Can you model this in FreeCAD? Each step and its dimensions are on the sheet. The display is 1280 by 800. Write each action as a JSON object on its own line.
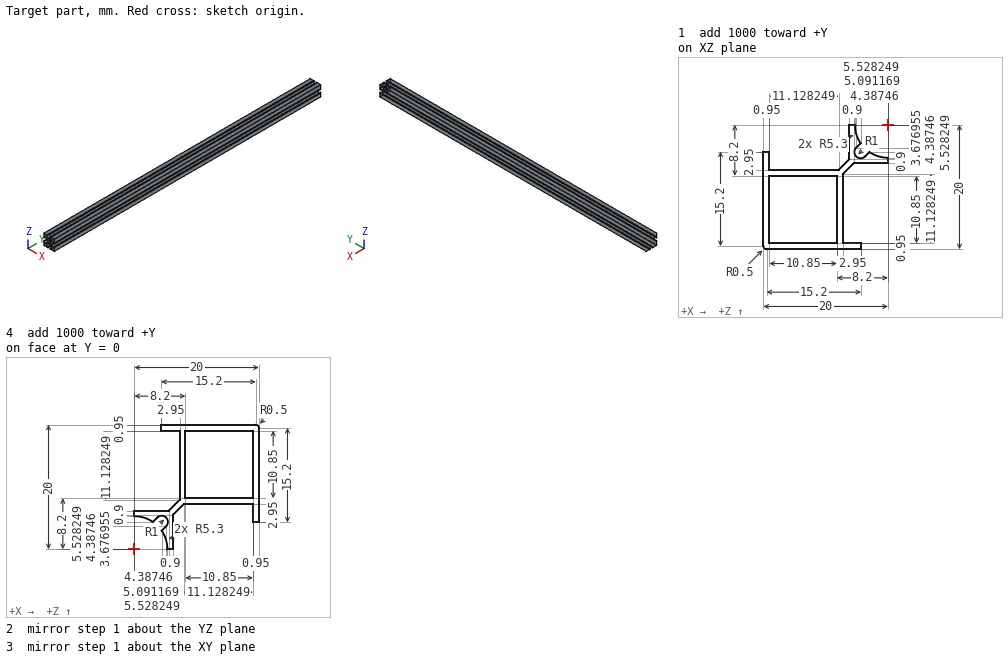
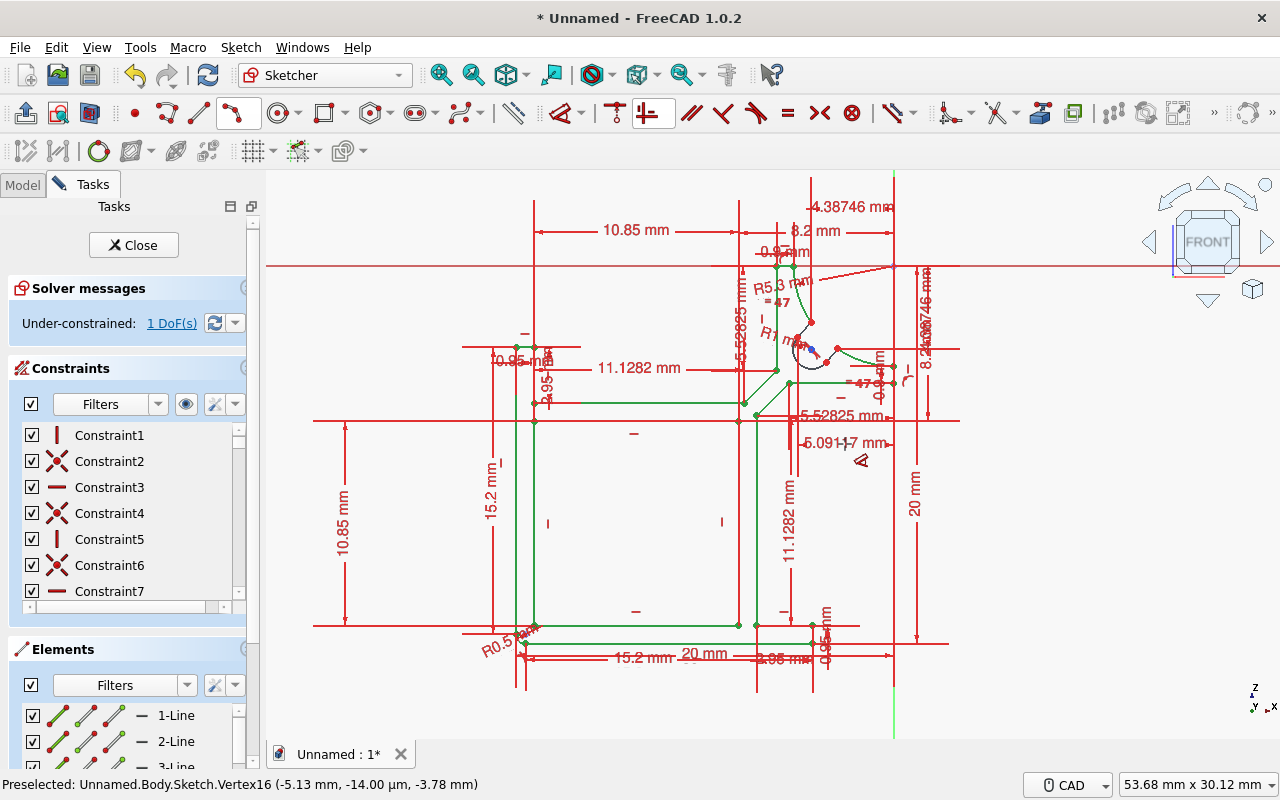
{"action": "left_click", "coordinate": [798, 338]}
{"action": "left_click", "coordinate": [928, 285]}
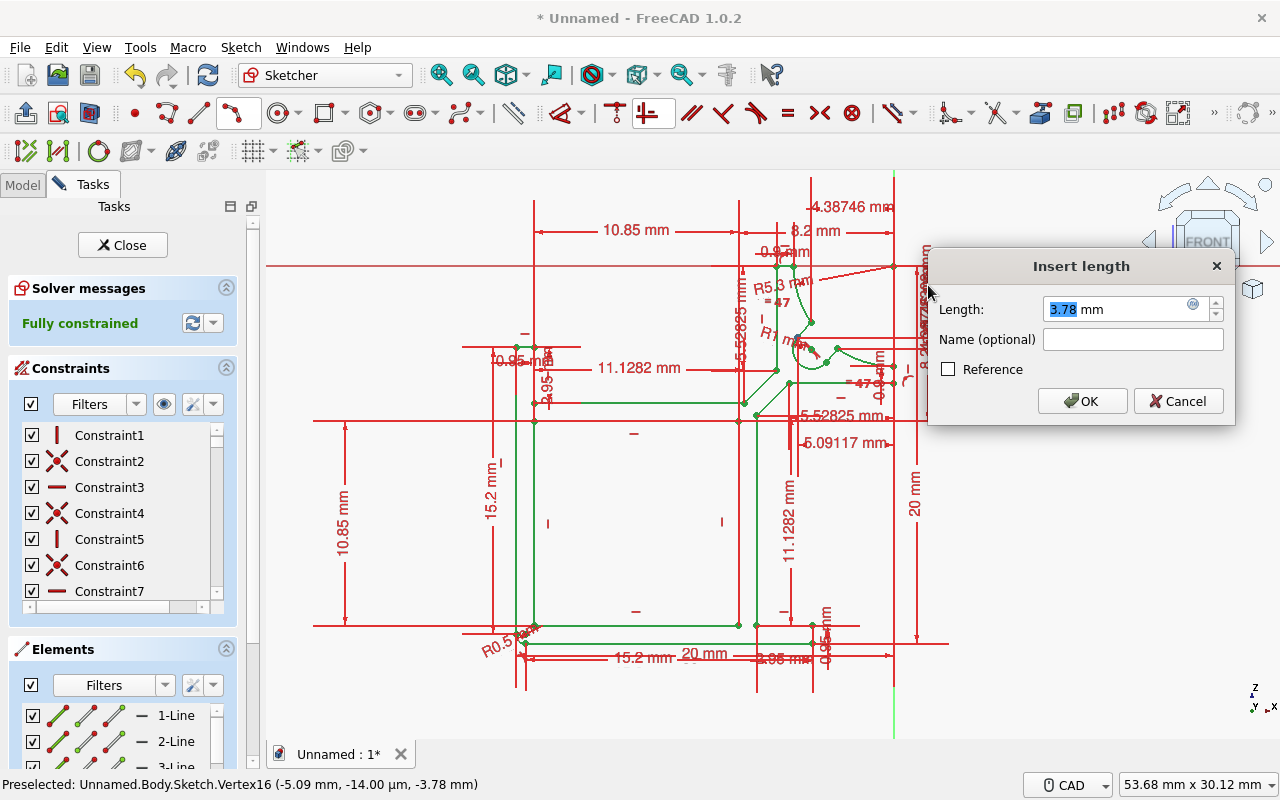
{"action": "type", "text": "3.676955"}
{"action": "key", "text": "Return"}
{"action": "key", "text": "Escape"}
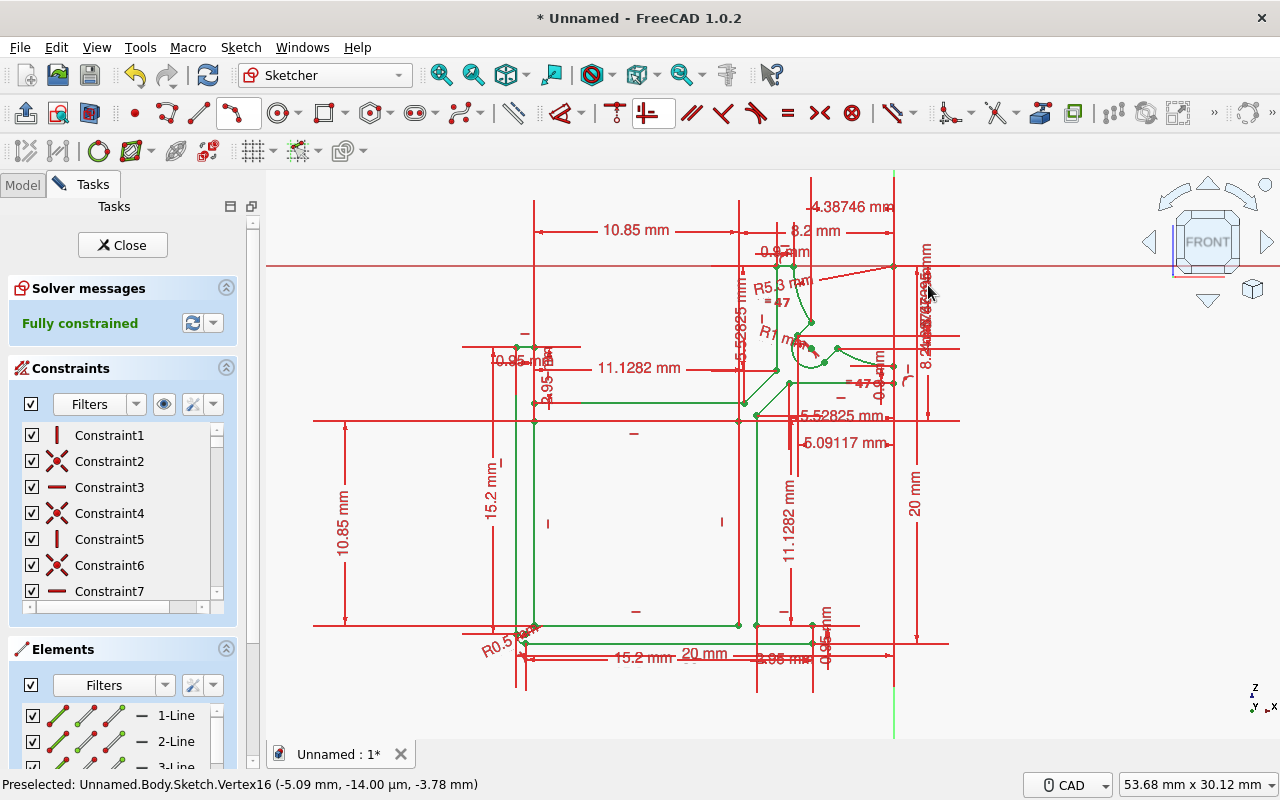
{"action": "left_click", "coordinate": [123, 245]}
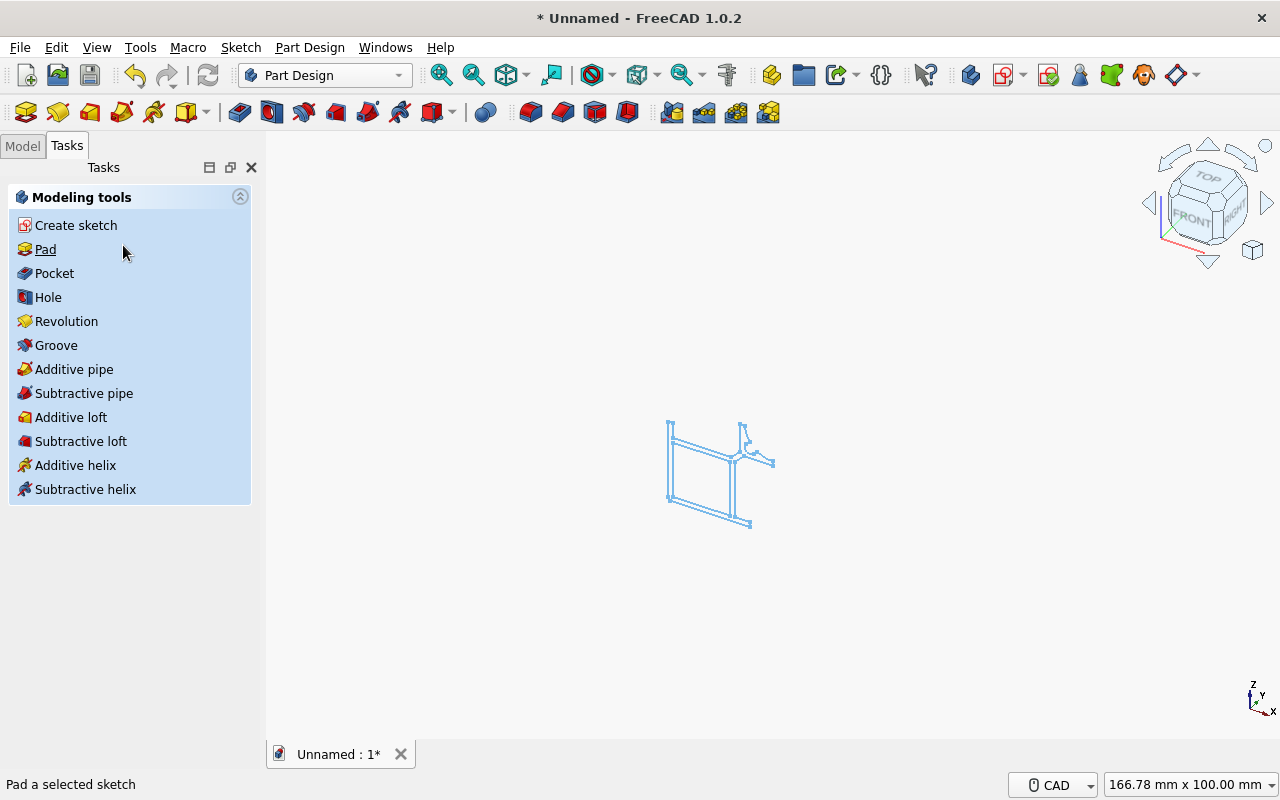
{"action": "left_click", "coordinate": [26, 112]}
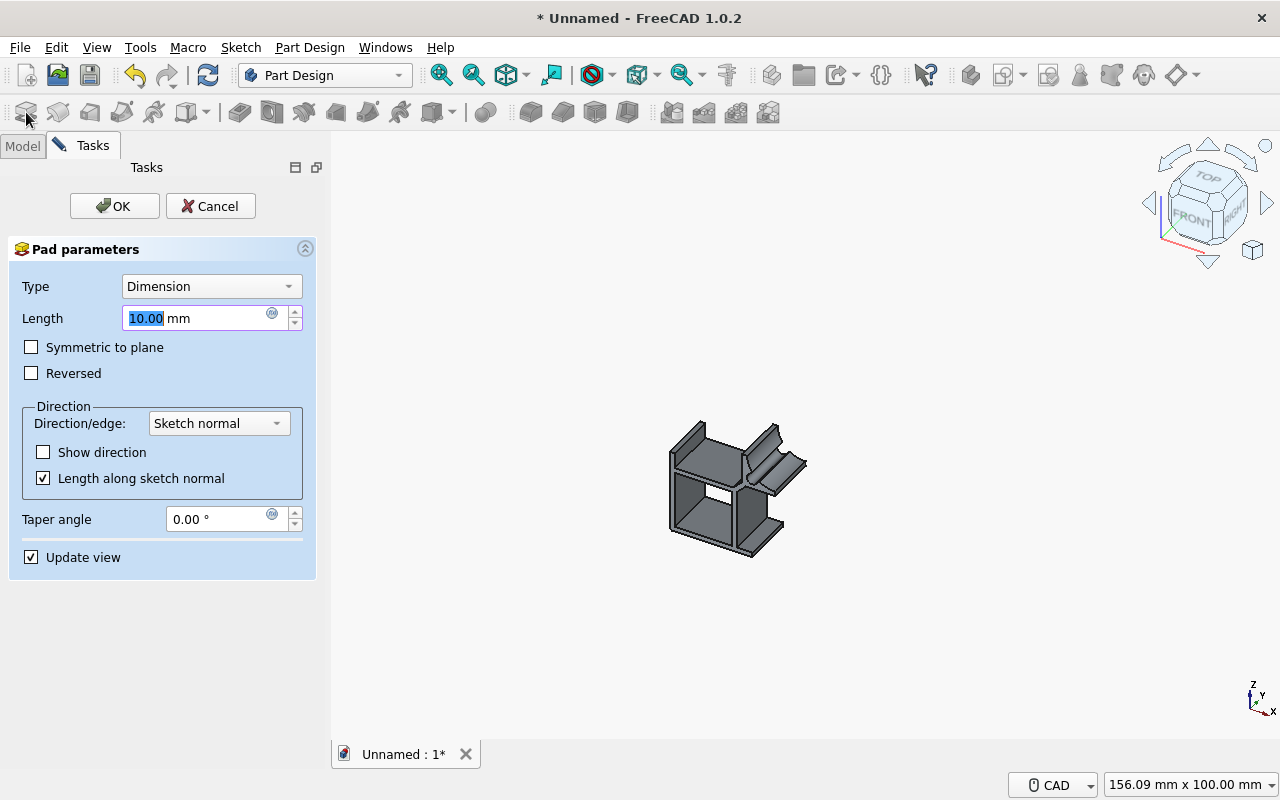
{"action": "type", "text": "1000"}
{"action": "key", "text": "Tab"}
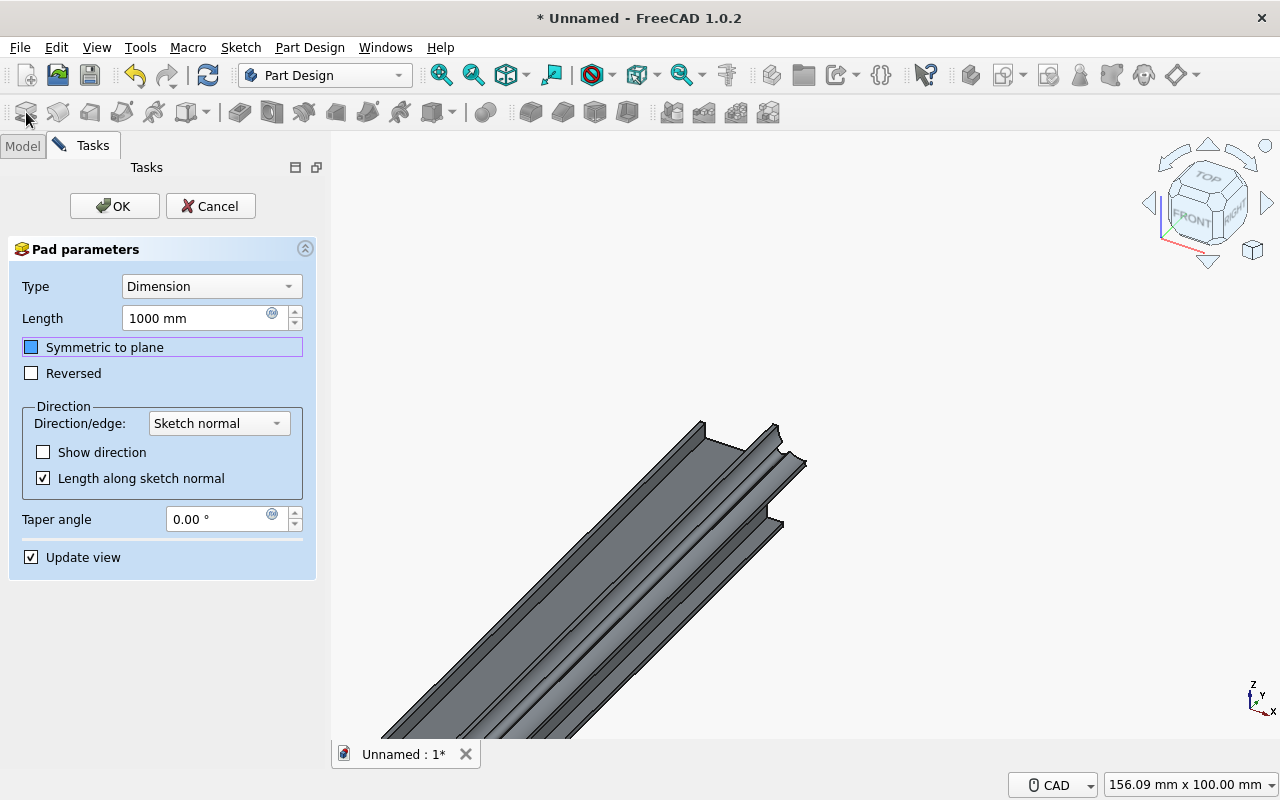
{"action": "left_click", "coordinate": [30, 373]}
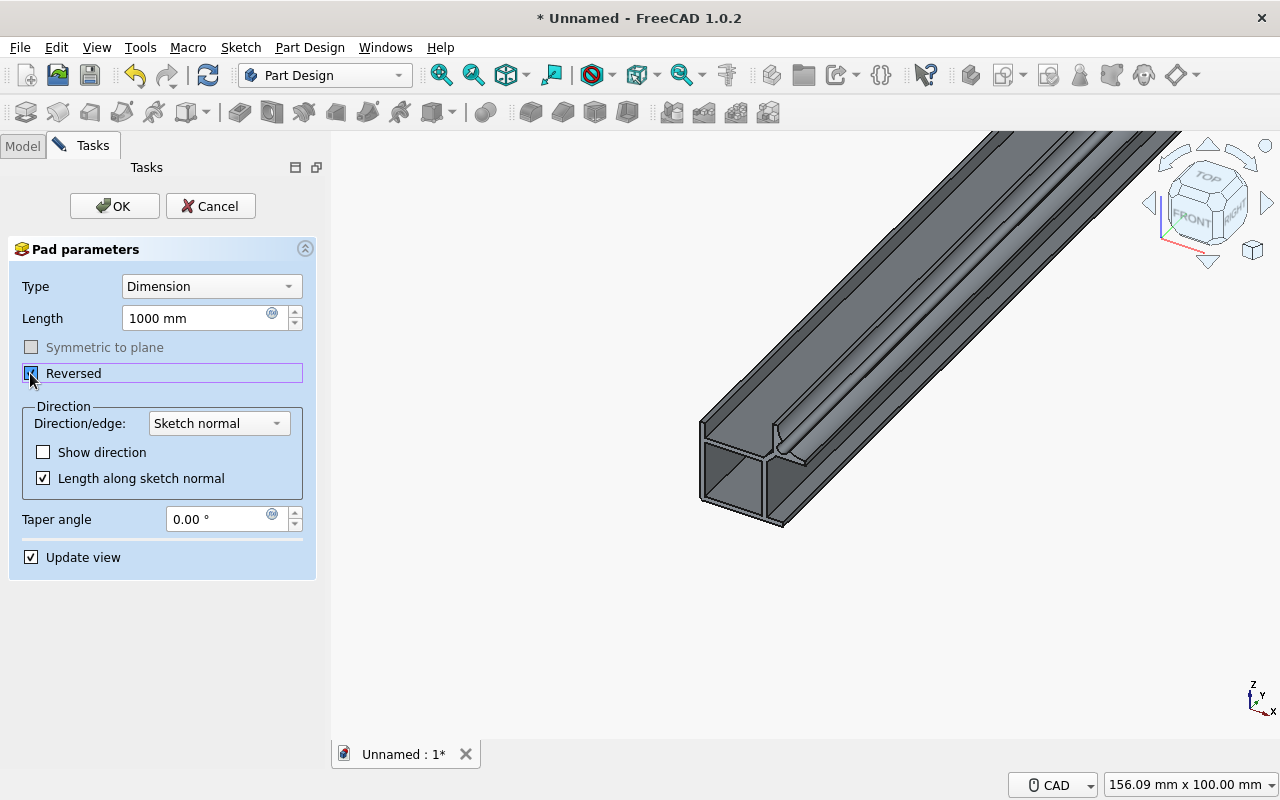
{"action": "left_click", "coordinate": [115, 206]}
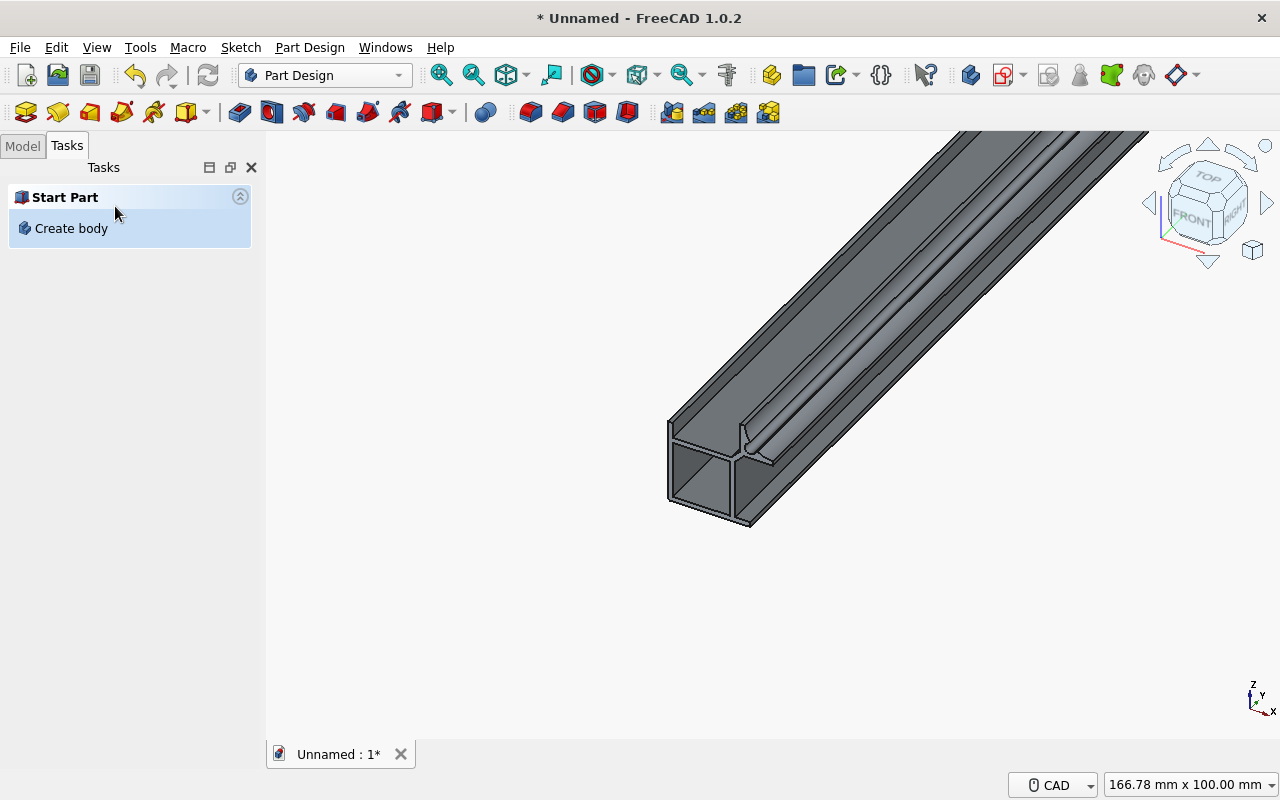
{"action": "left_click", "coordinate": [442, 76]}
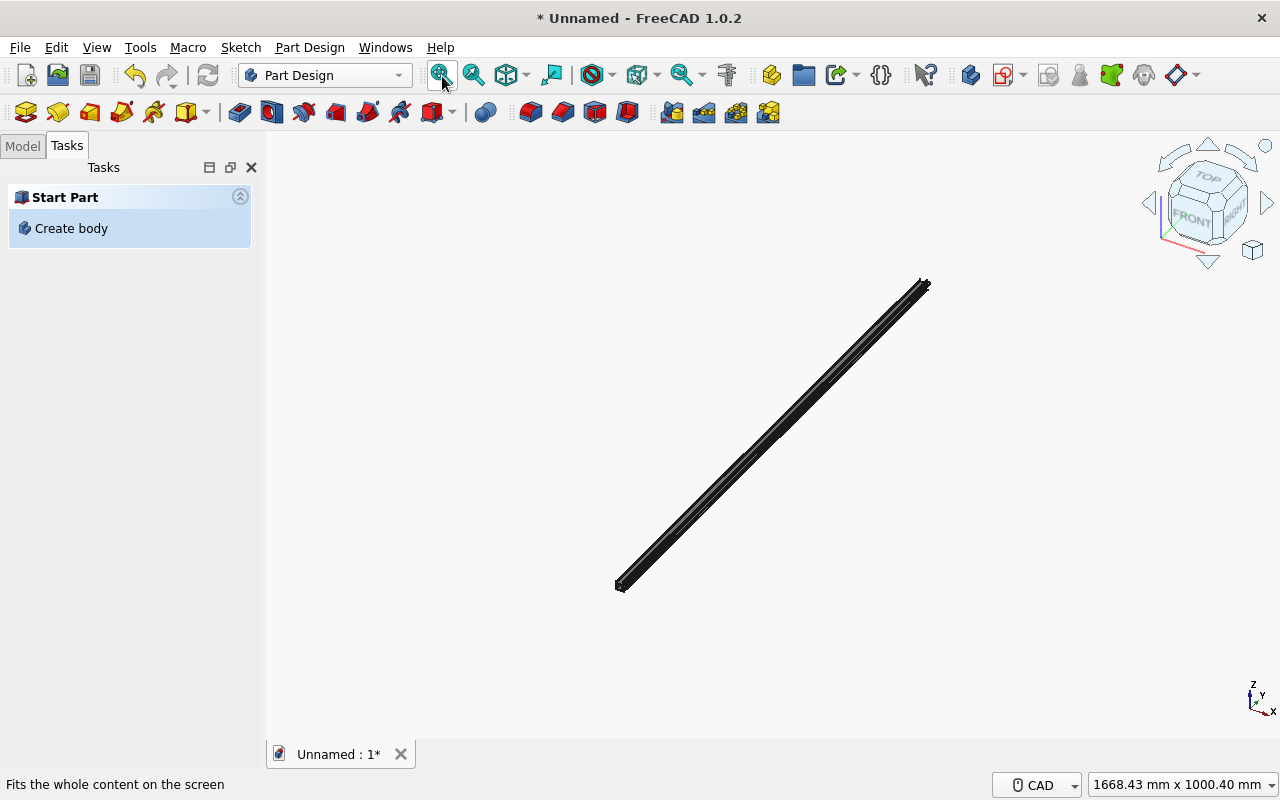
{"action": "left_click", "coordinate": [23, 145]}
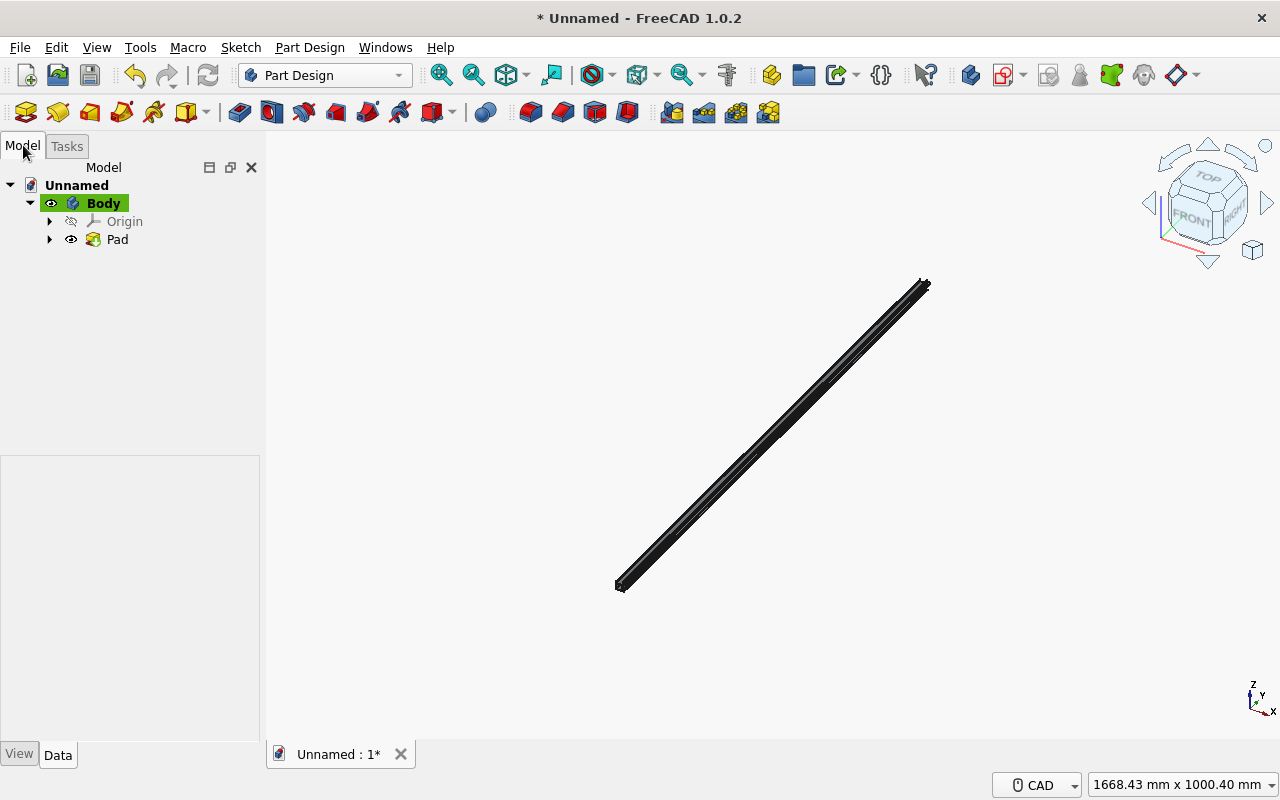
{"action": "left_click", "coordinate": [116, 239]}